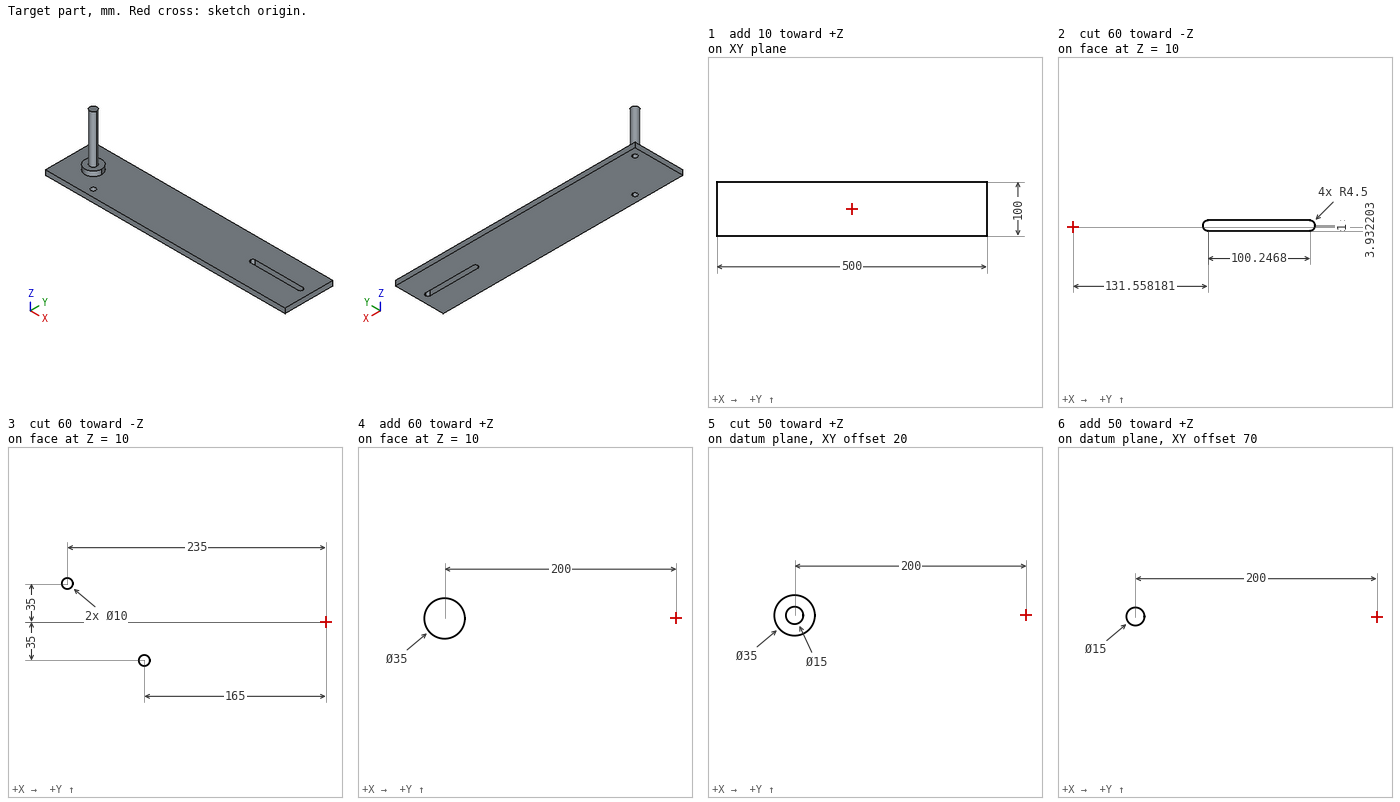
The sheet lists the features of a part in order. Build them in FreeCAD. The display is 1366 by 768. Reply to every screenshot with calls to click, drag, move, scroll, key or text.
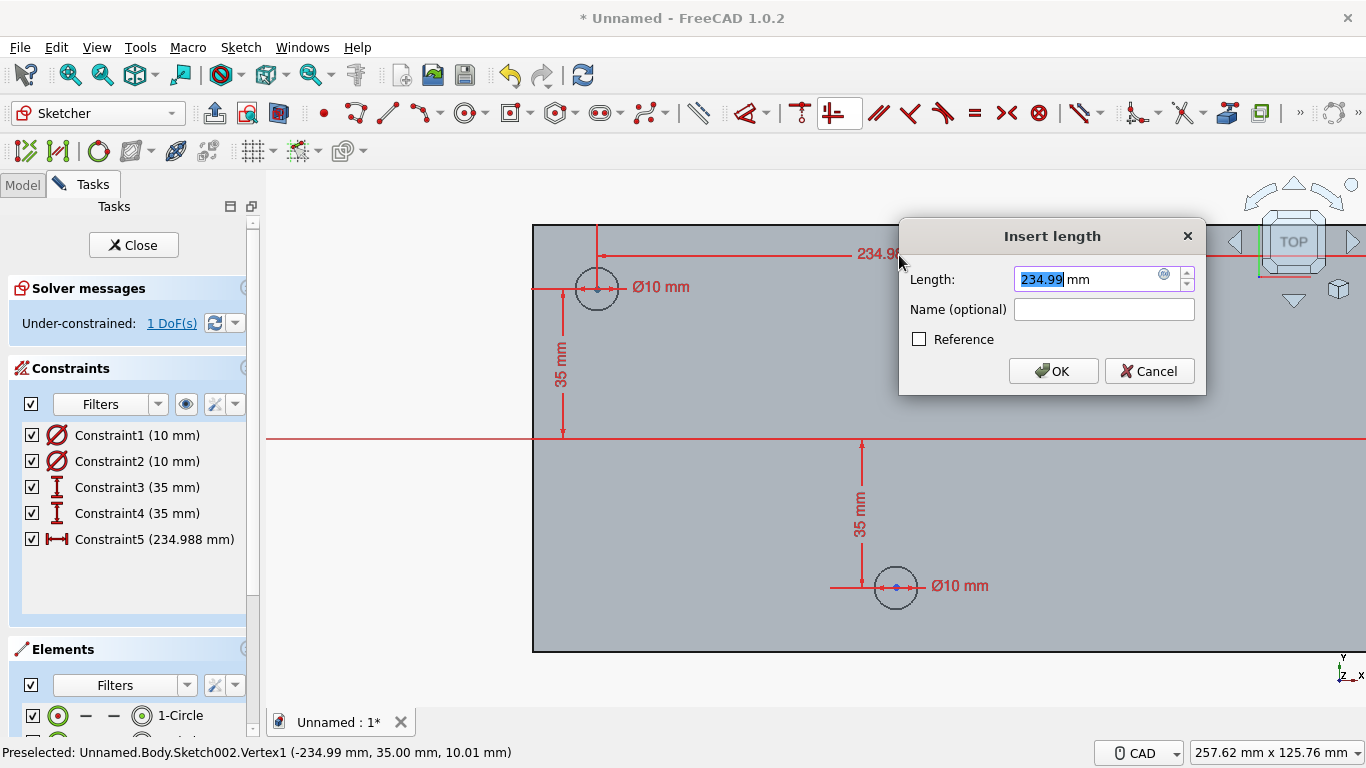
text(235)
key(Return)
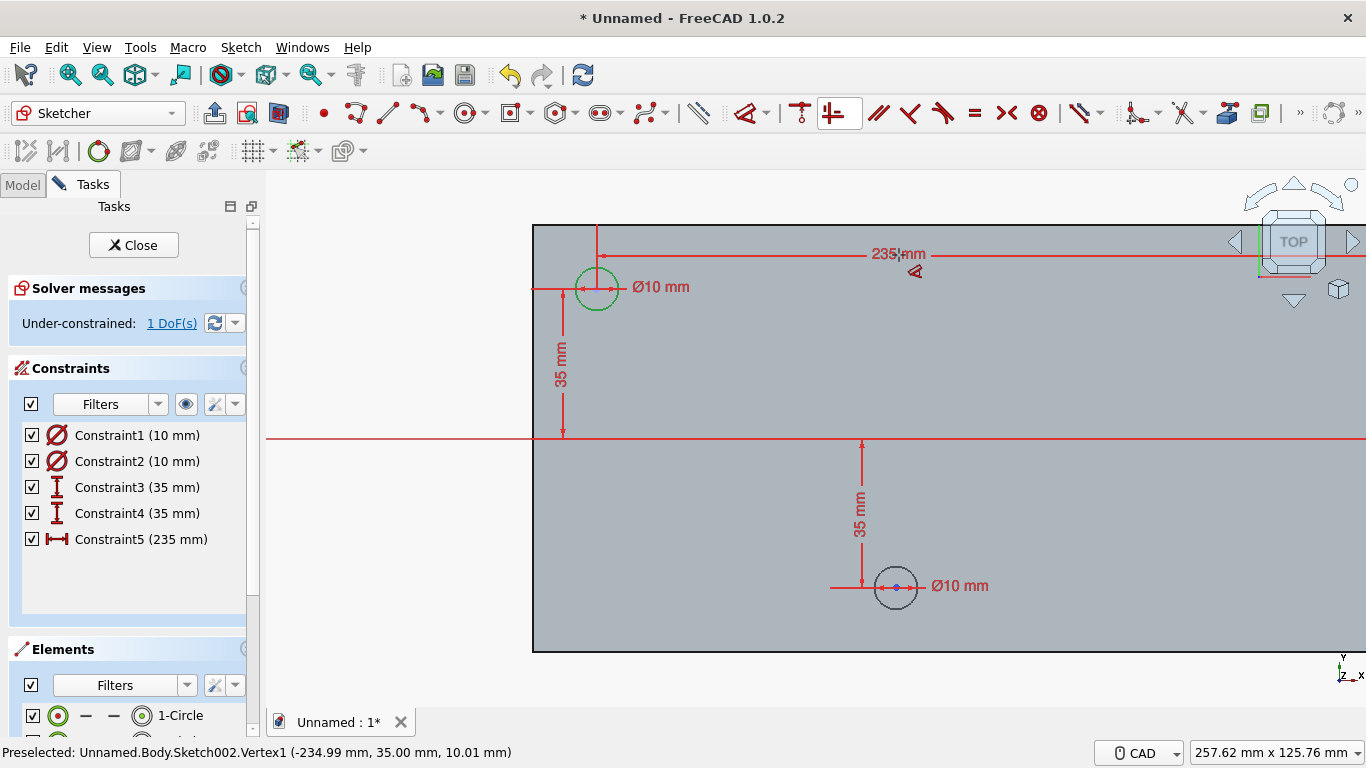
click(896, 588)
click(1048, 622)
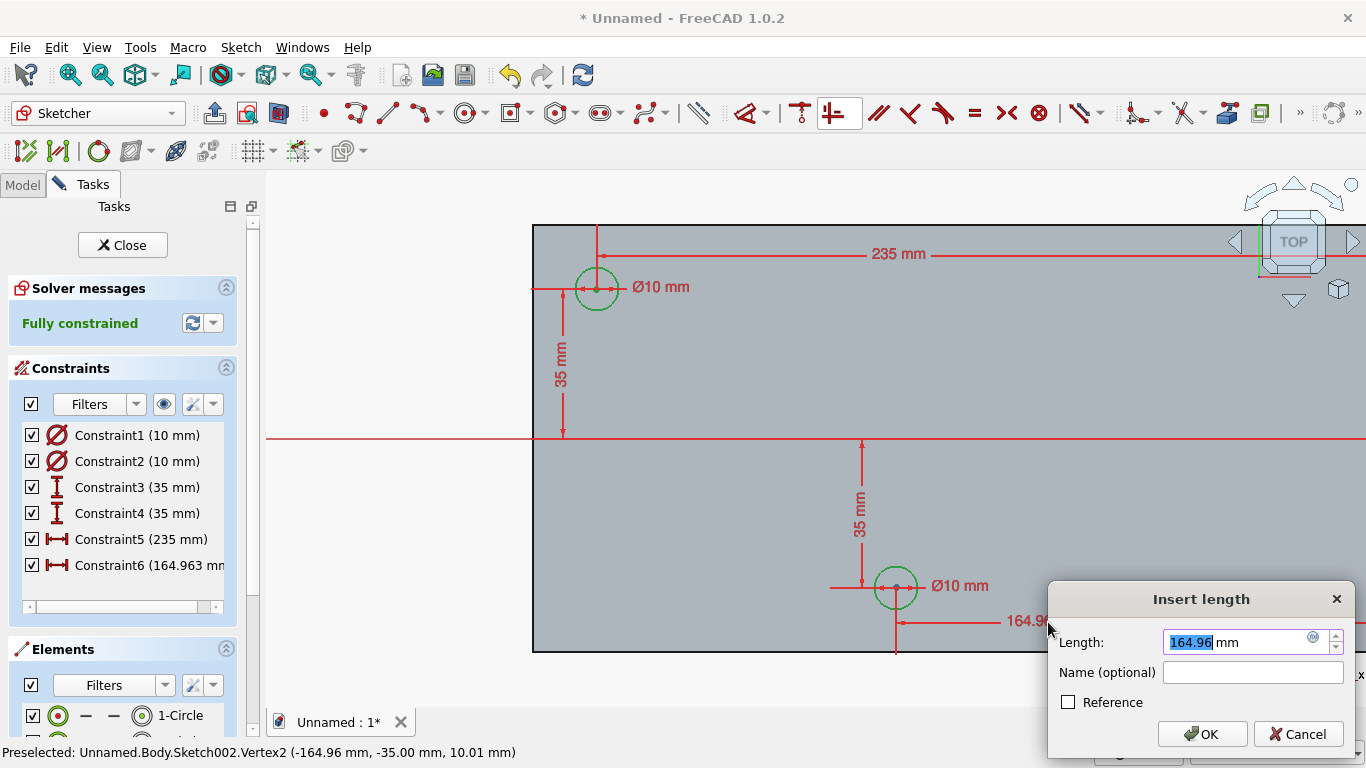
text(165)
key(Return)
key(Escape)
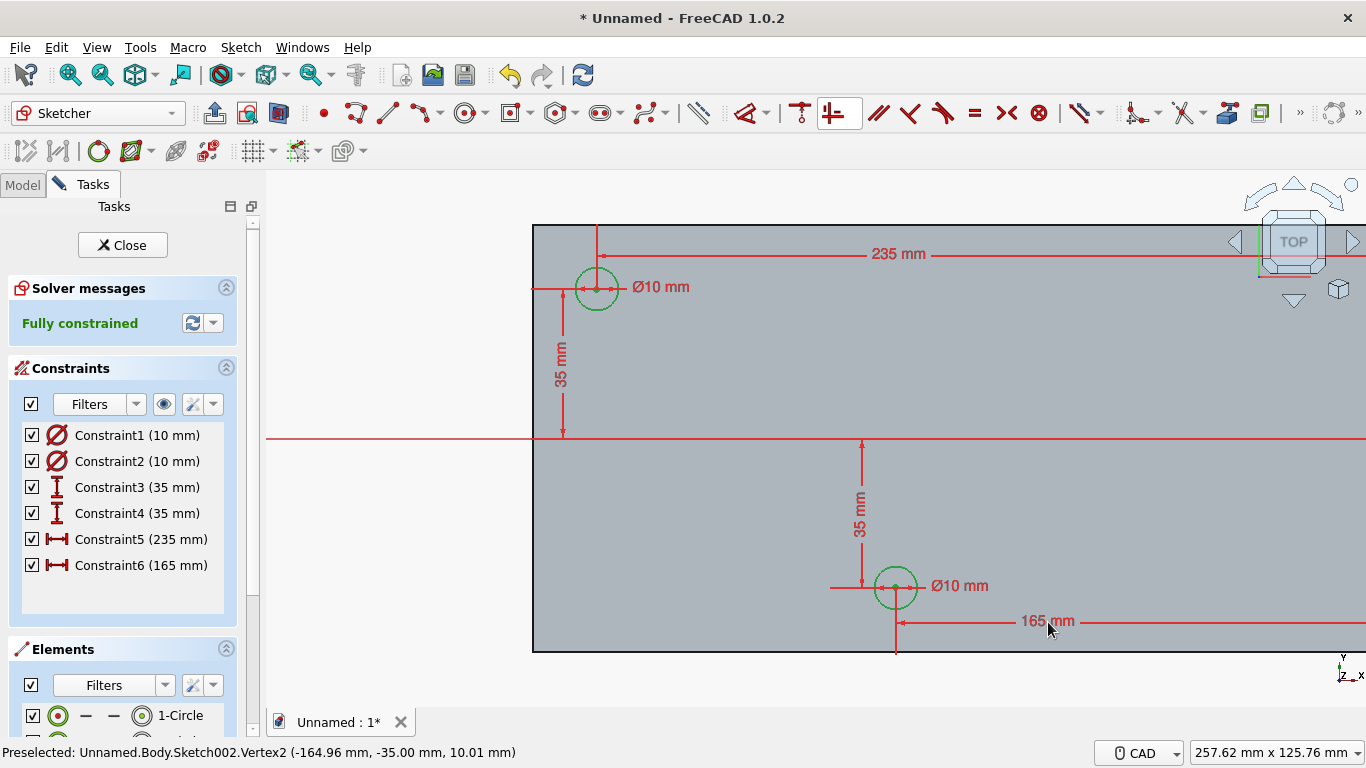
click(123, 245)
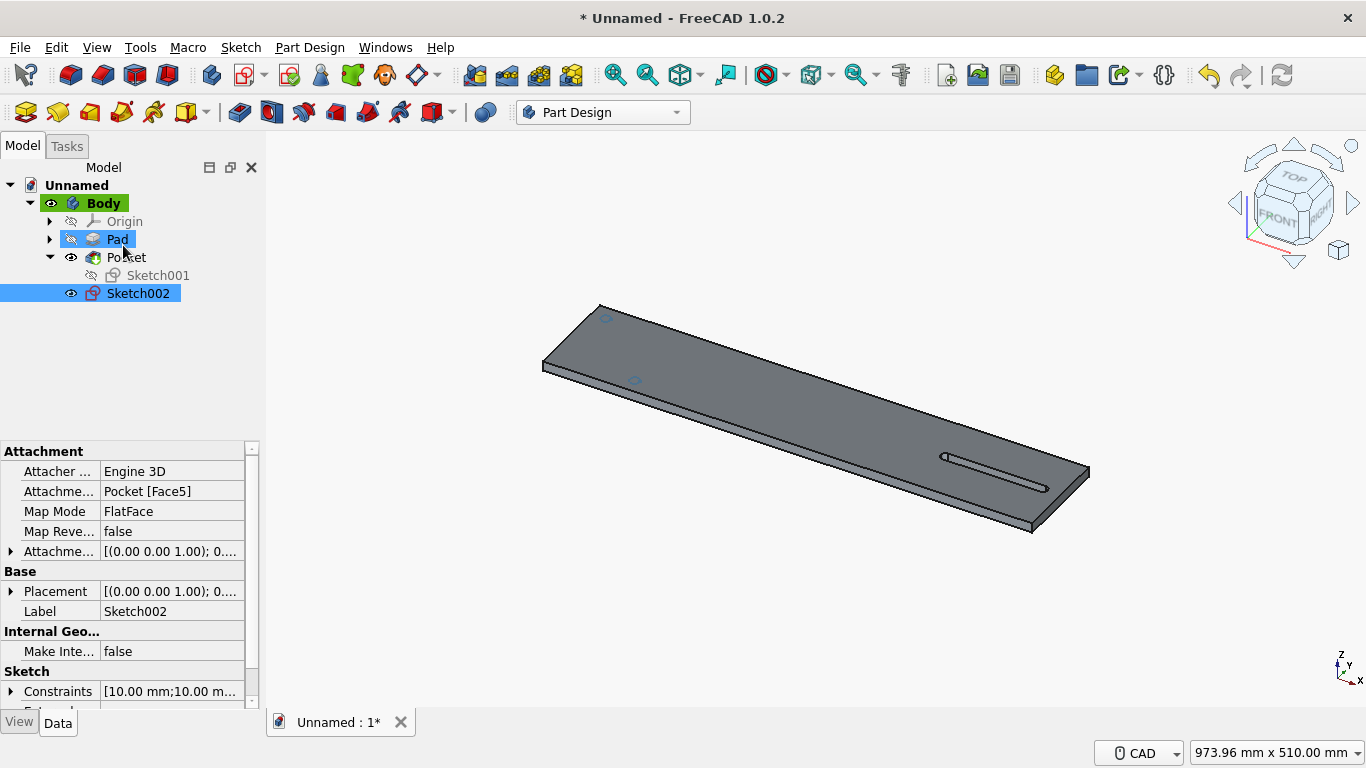
click(240, 112)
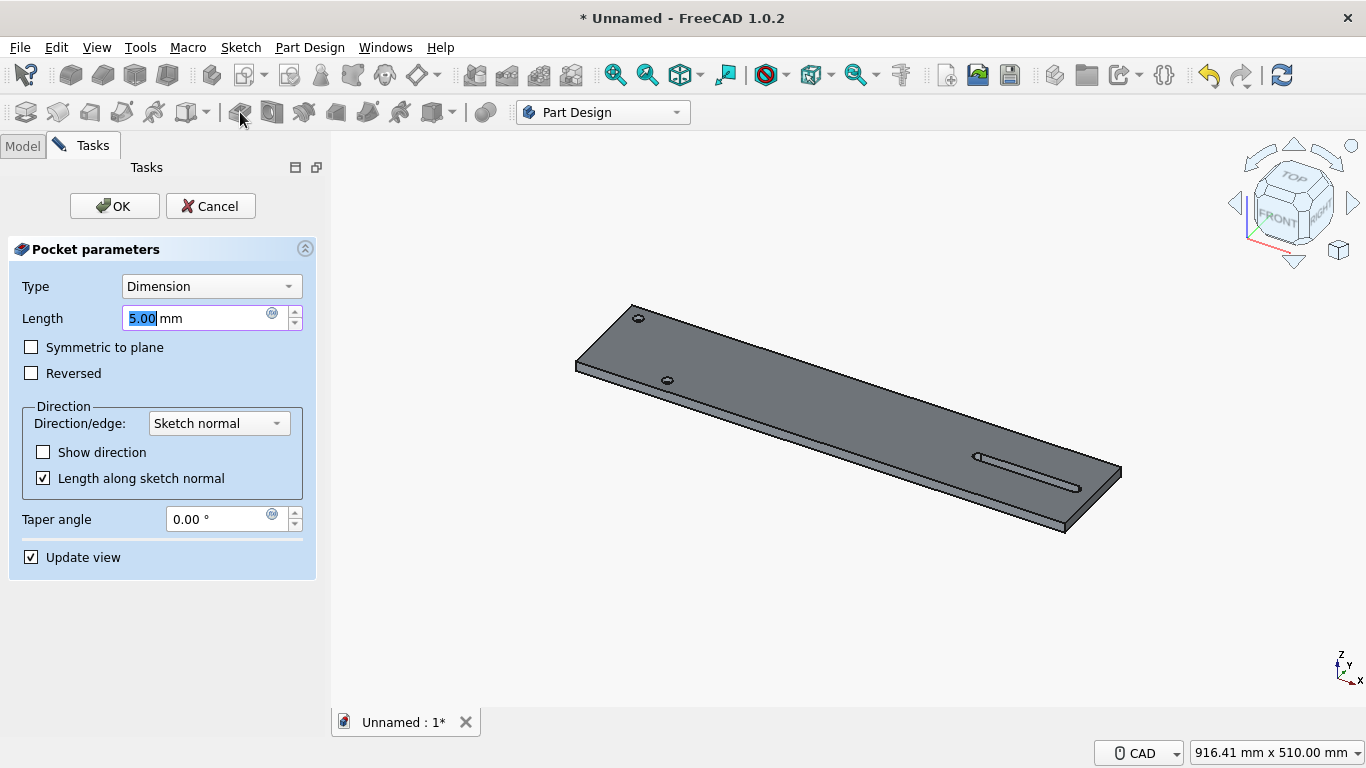
text(60)
key(Tab)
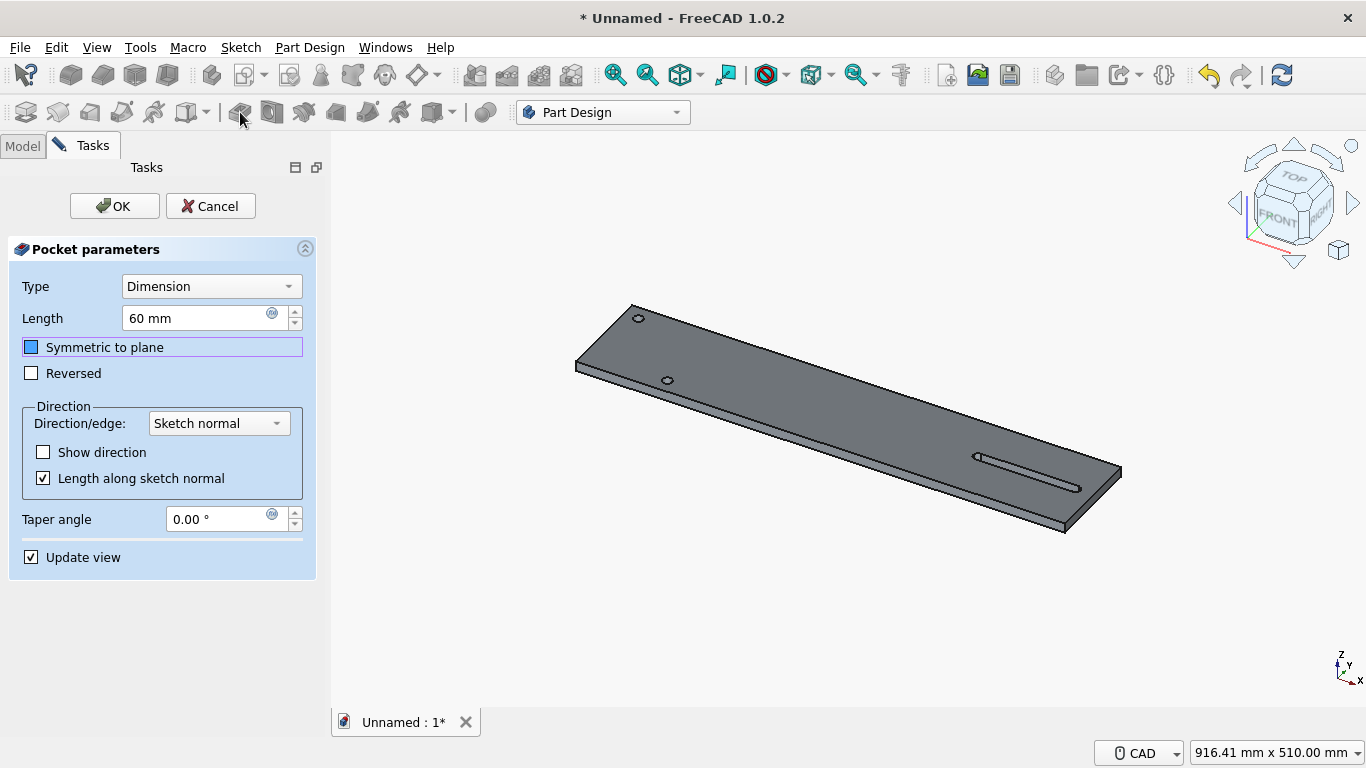
click(115, 206)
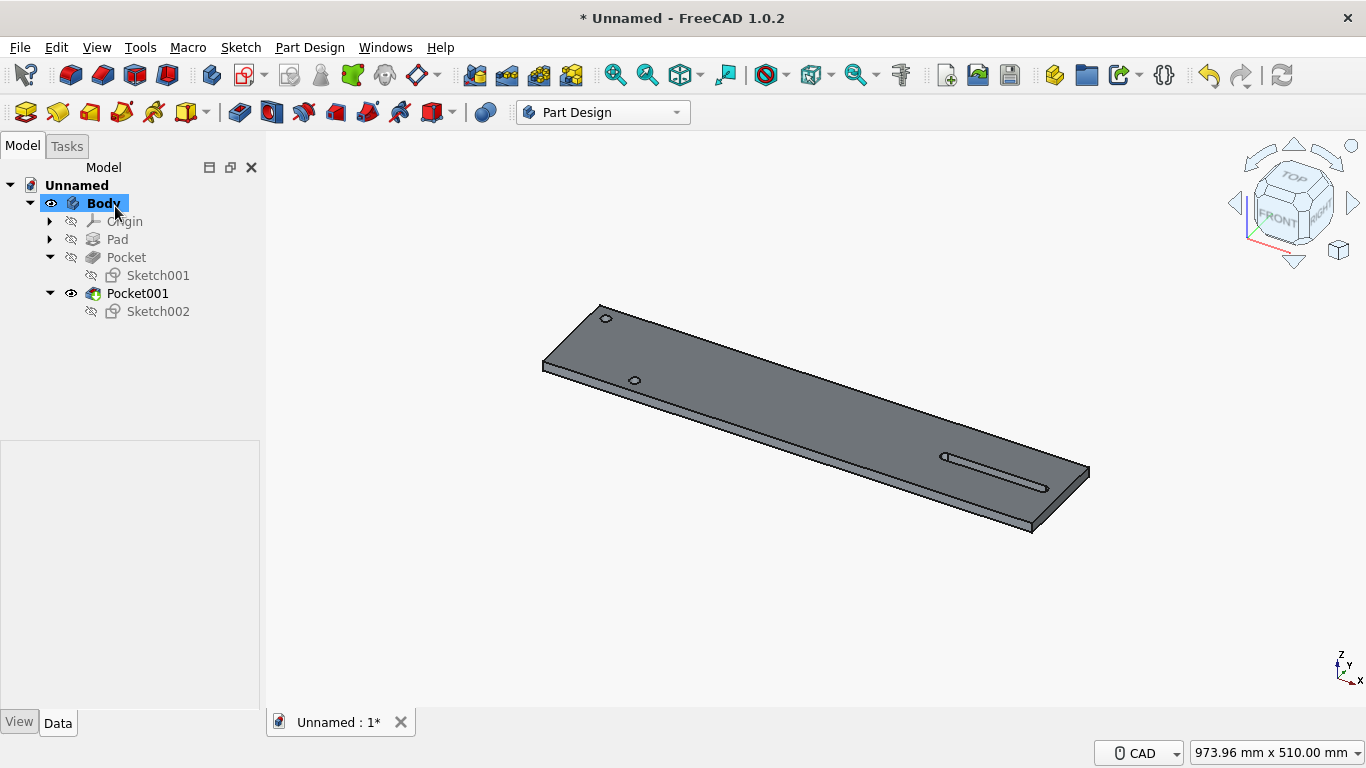
click(886, 437)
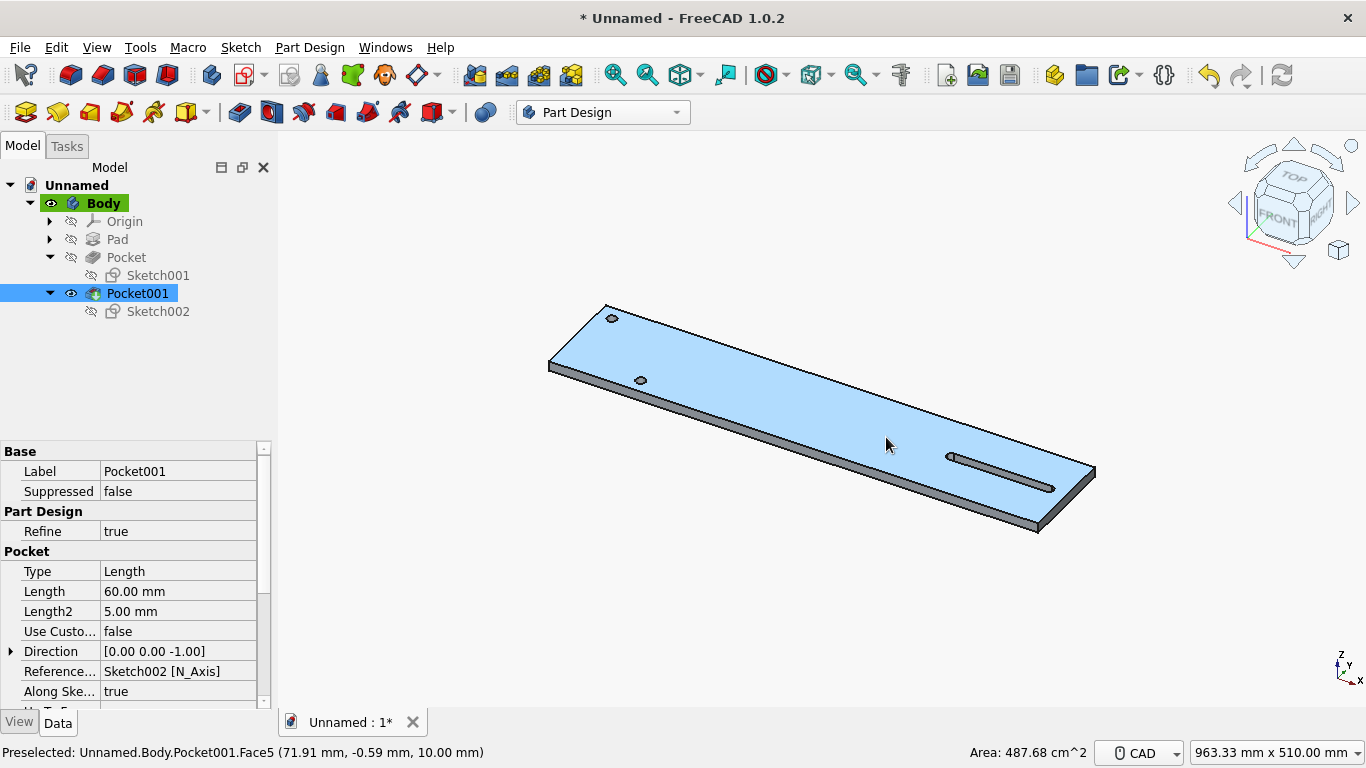
click(244, 76)